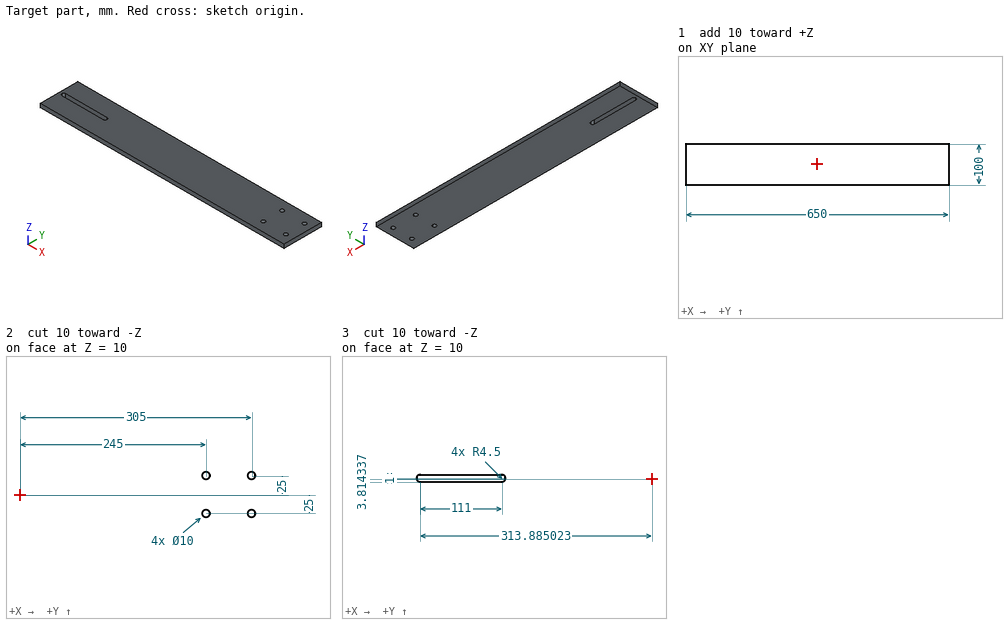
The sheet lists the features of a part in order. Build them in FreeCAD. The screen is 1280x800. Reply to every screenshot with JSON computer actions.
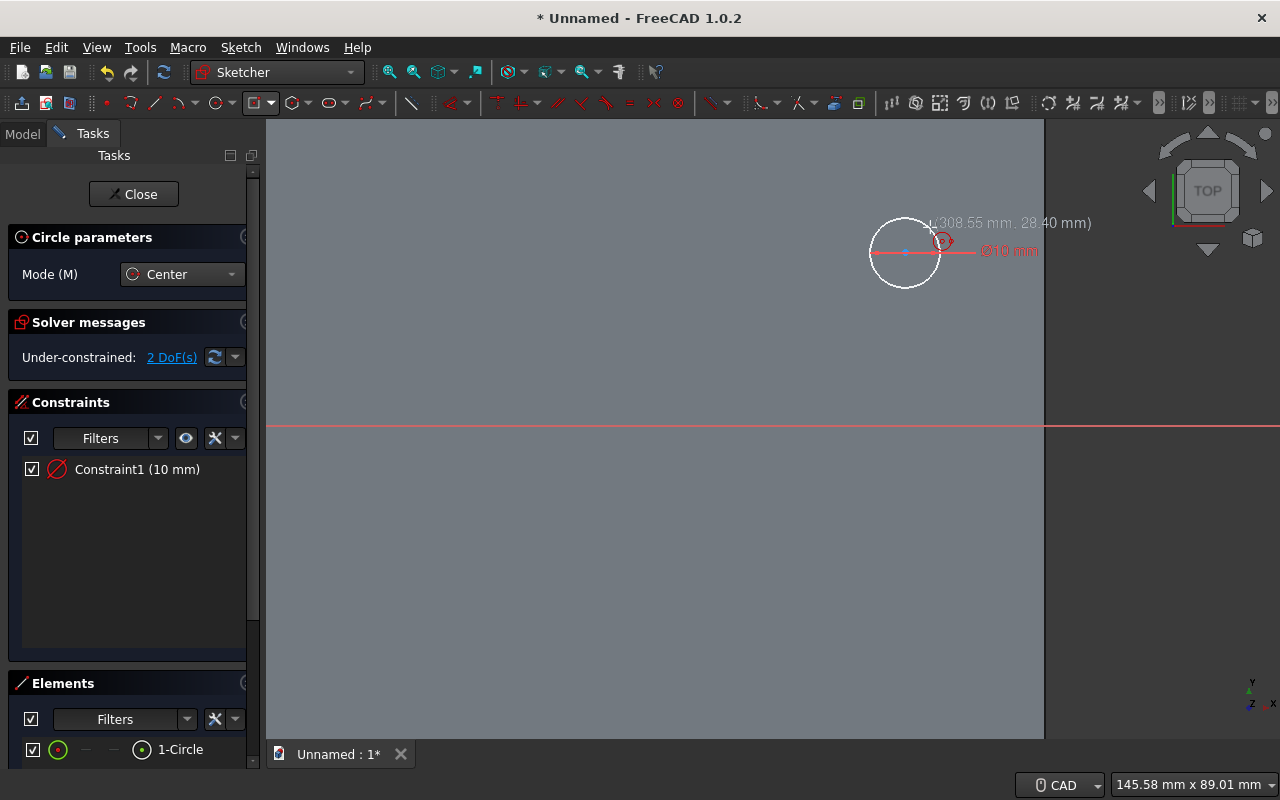
{"action": "left_click", "coordinate": [487, 252]}
{"action": "mouse_move", "coordinate": [512, 227]}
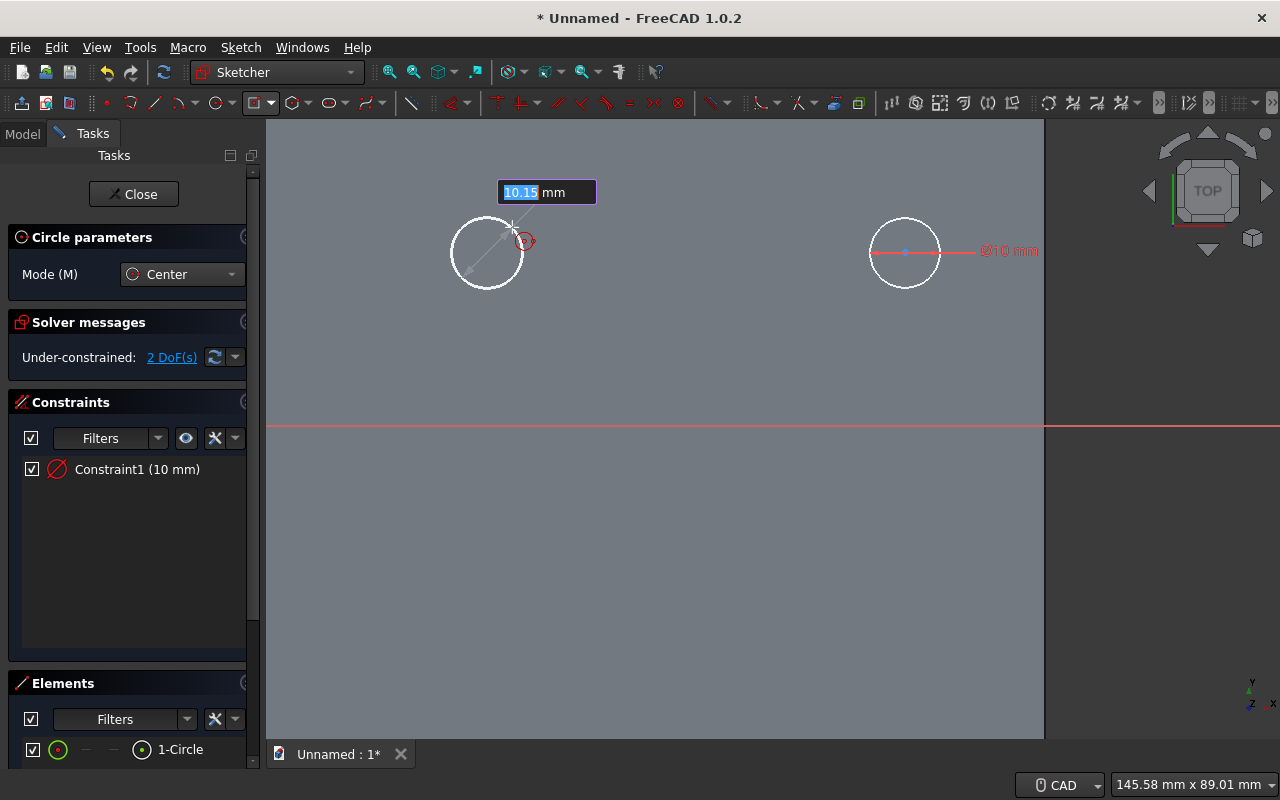
{"action": "type", "text": "10"}
{"action": "key", "text": "Return"}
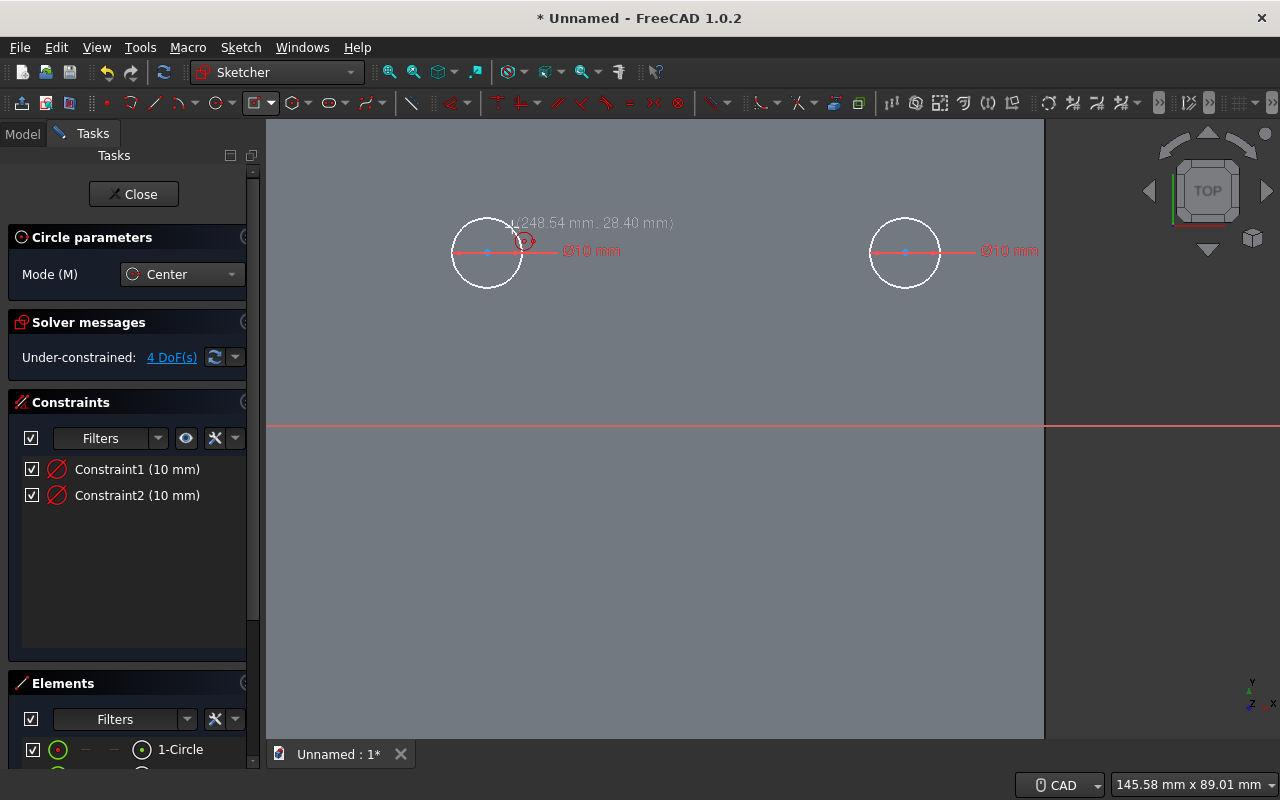
{"action": "left_click", "coordinate": [487, 600]}
{"action": "mouse_move", "coordinate": [512, 575]}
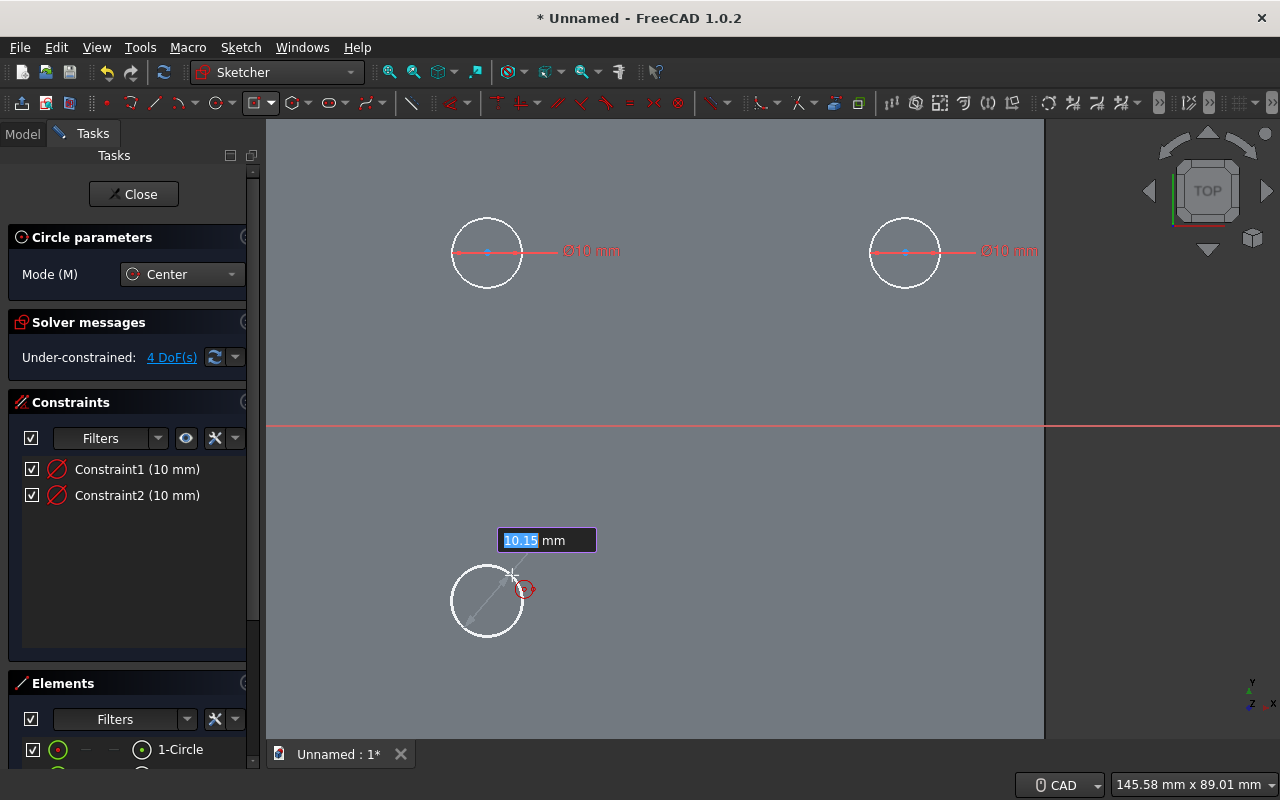
{"action": "type", "text": "10"}
{"action": "key", "text": "Return"}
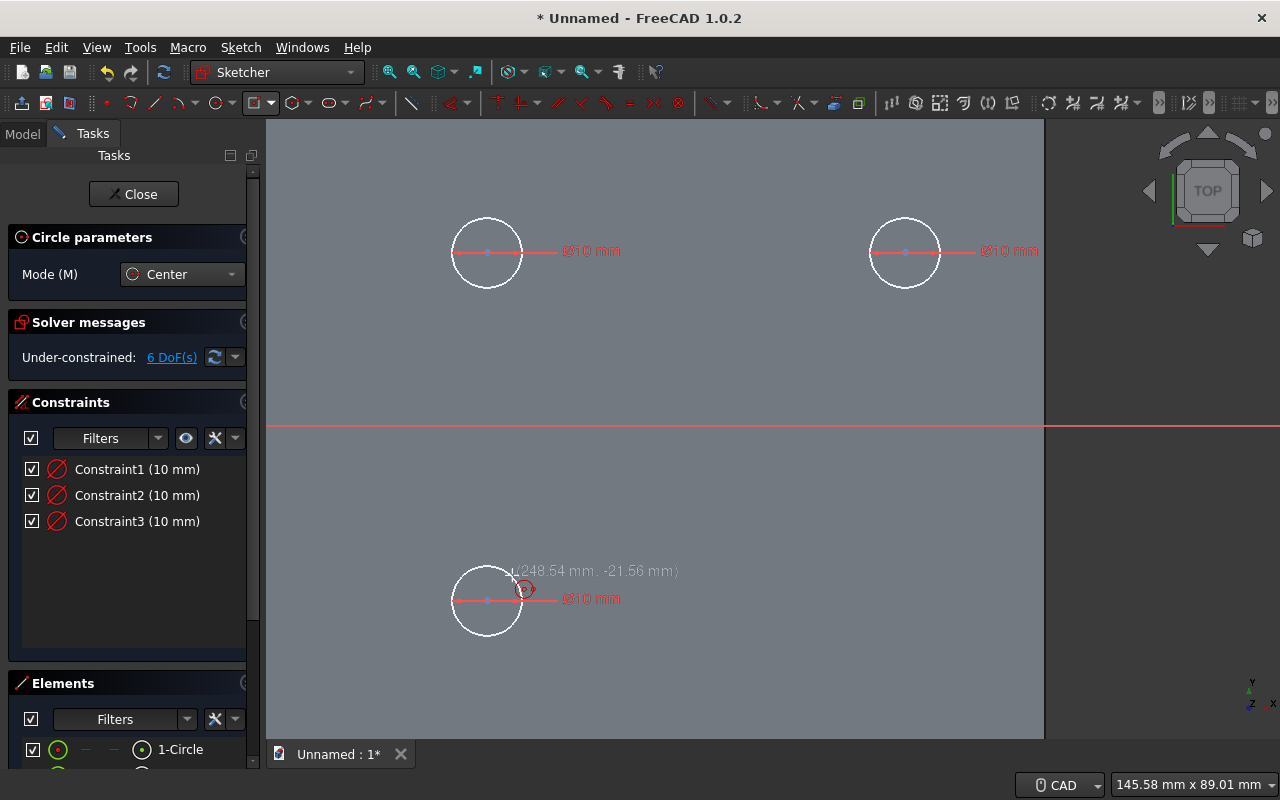
{"action": "left_click", "coordinate": [905, 600]}
{"action": "mouse_move", "coordinate": [930, 575]}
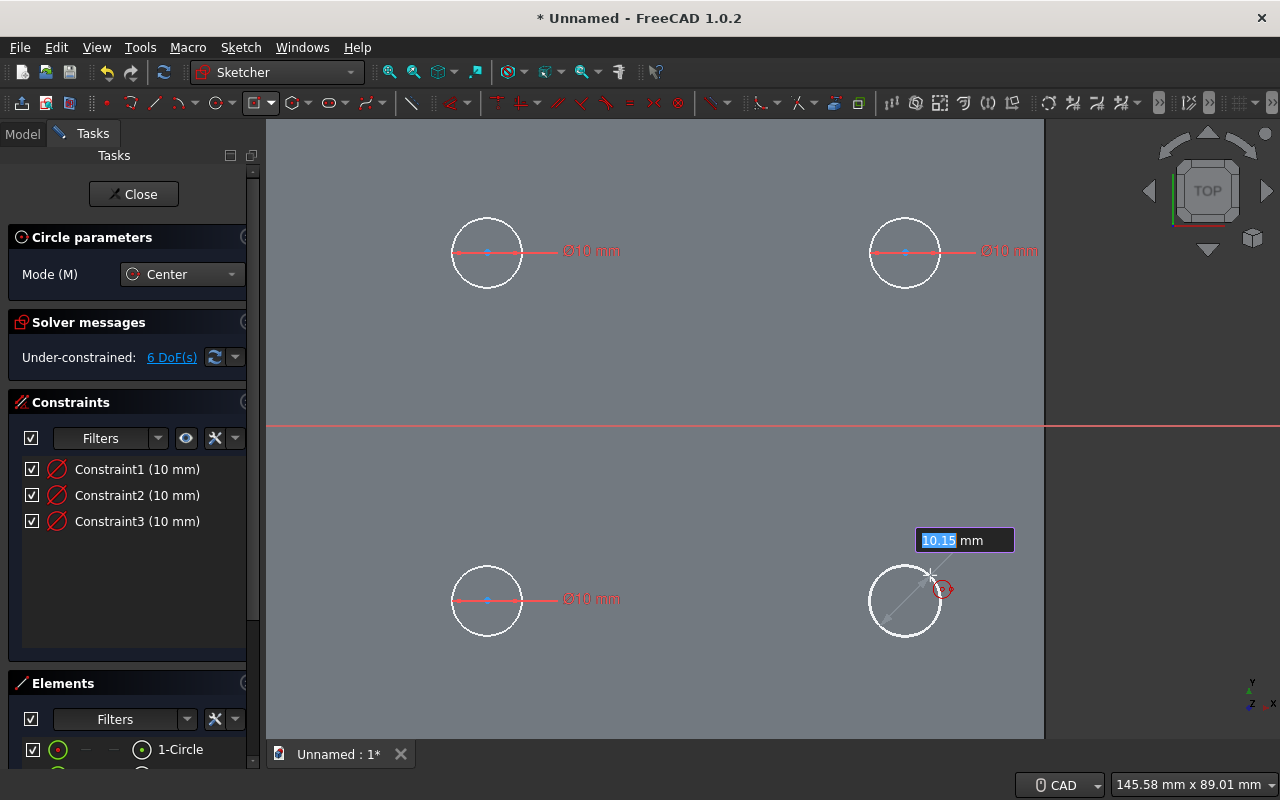
{"action": "type", "text": "10"}
{"action": "key", "text": "Return"}
{"action": "key", "text": "Escape"}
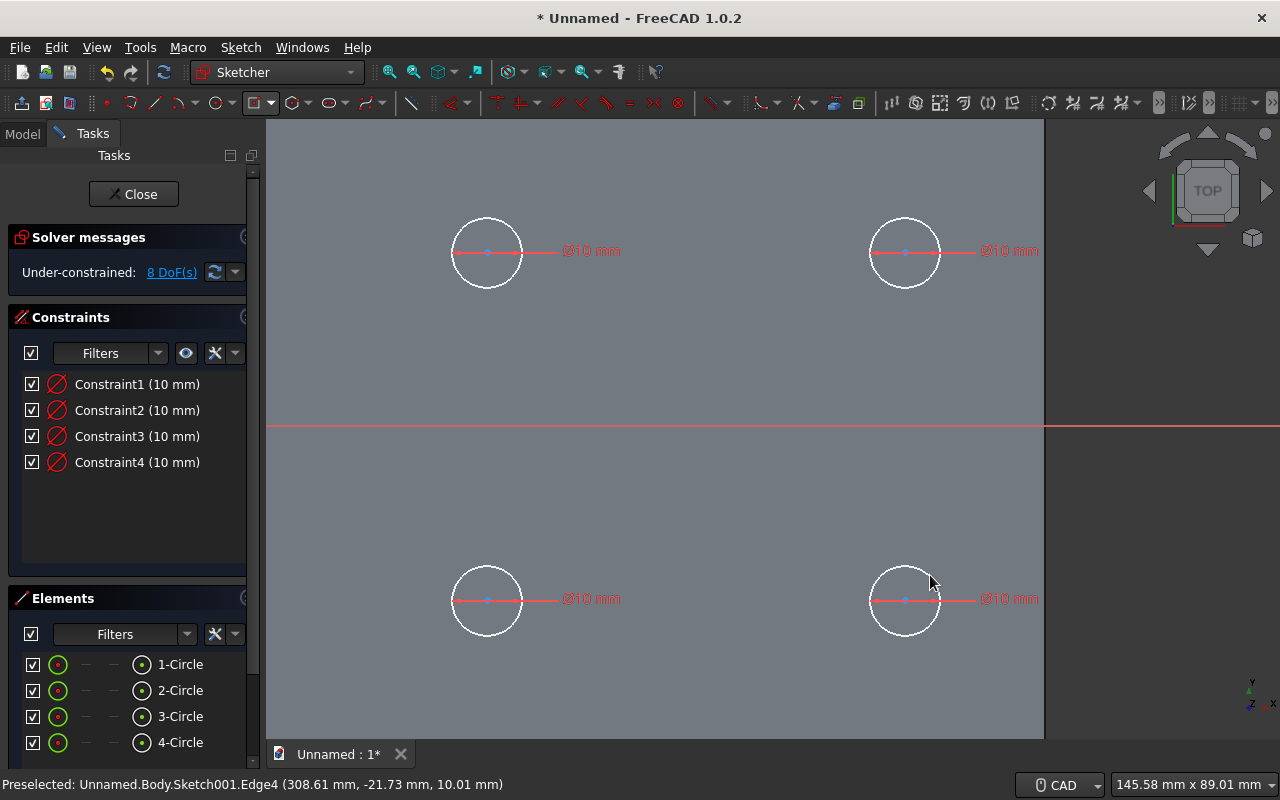
{"action": "left_click", "coordinate": [905, 253]}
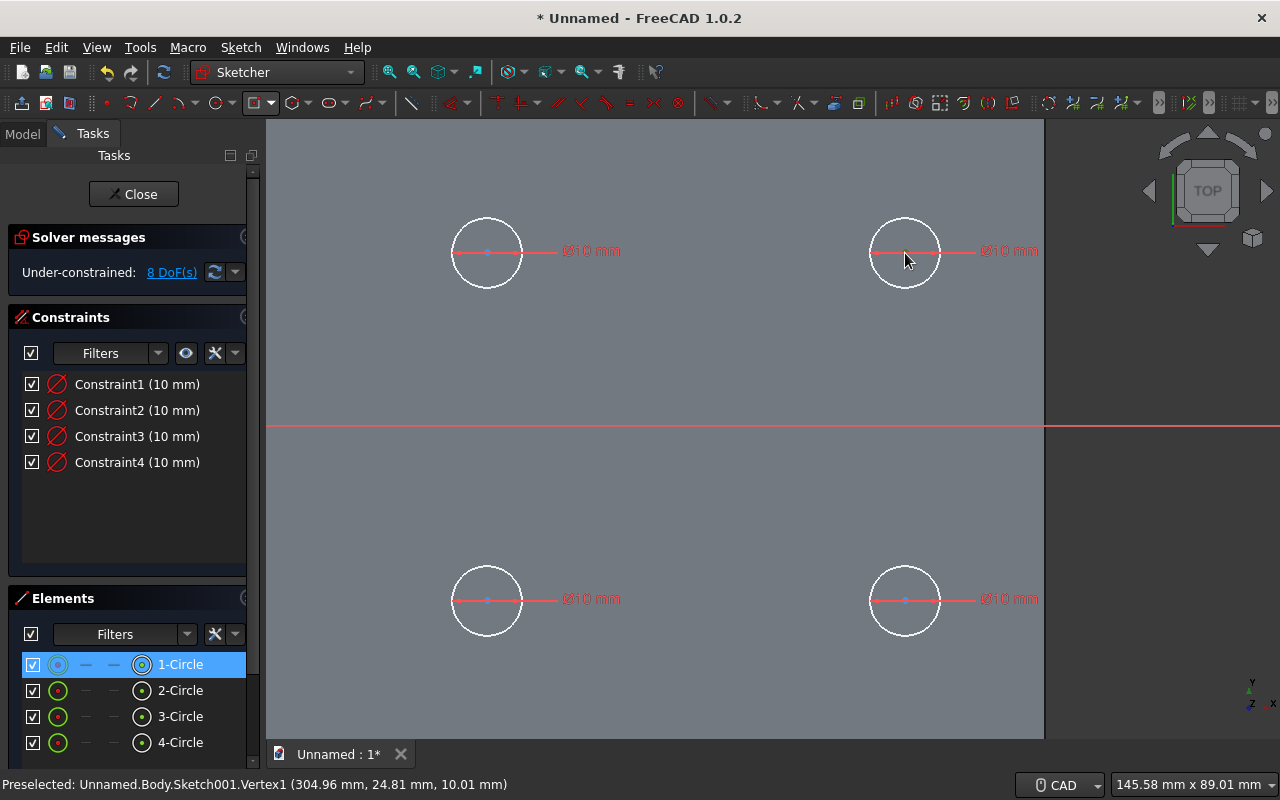
{"action": "left_click", "coordinate": [487, 253]}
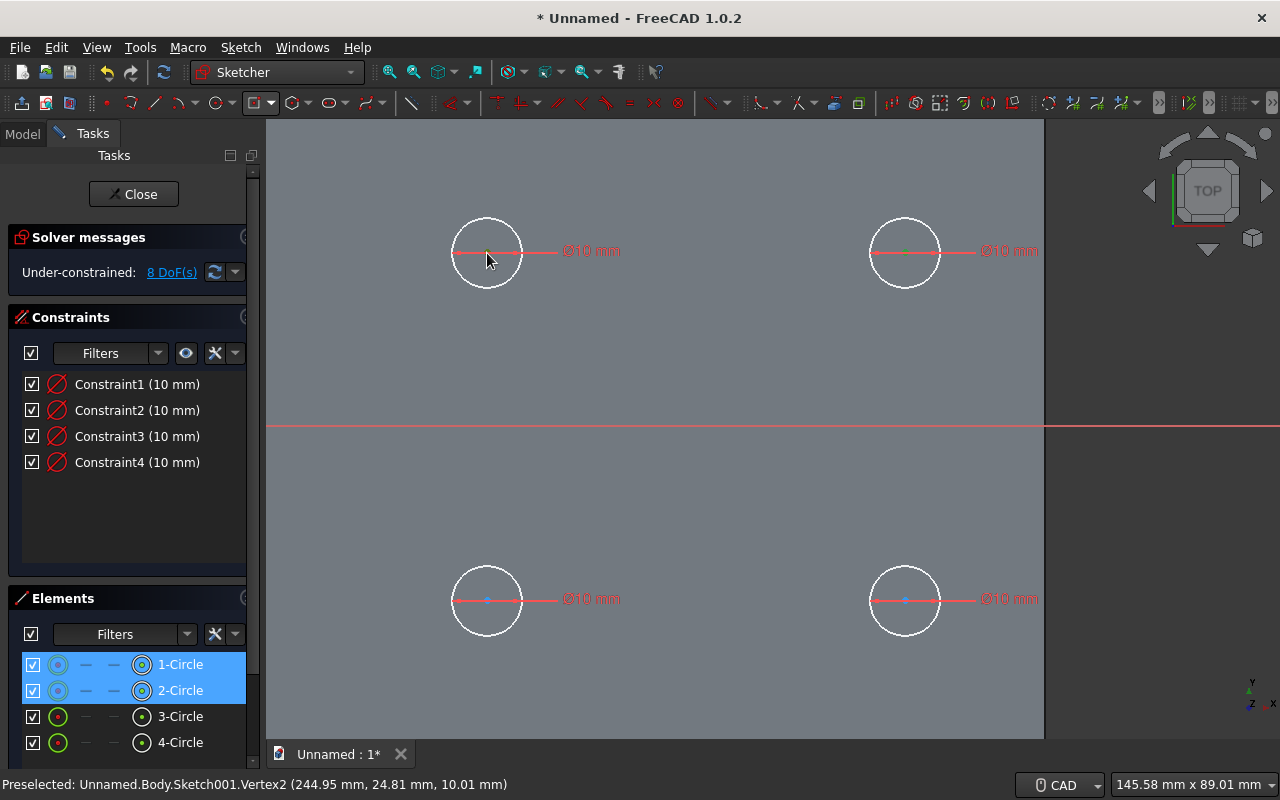
{"action": "key", "text": "h"}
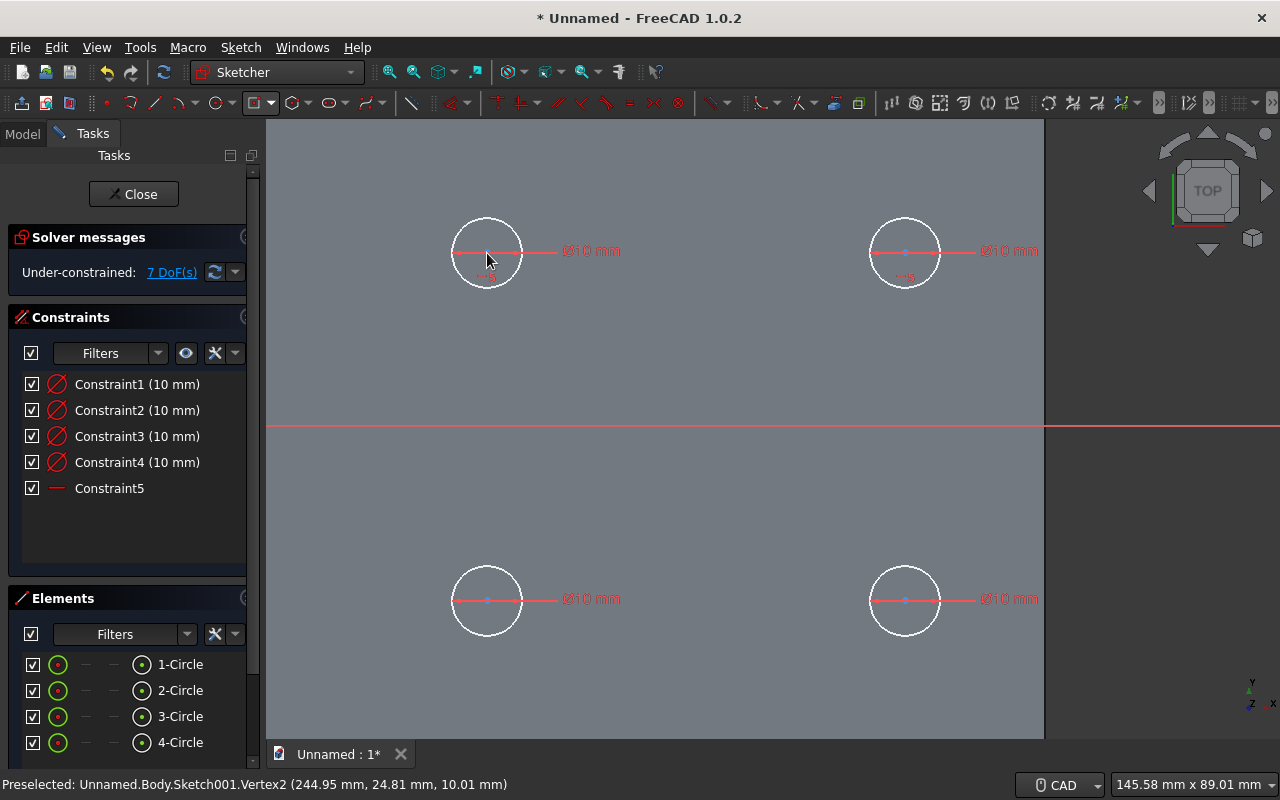
{"action": "left_click", "coordinate": [487, 253]}